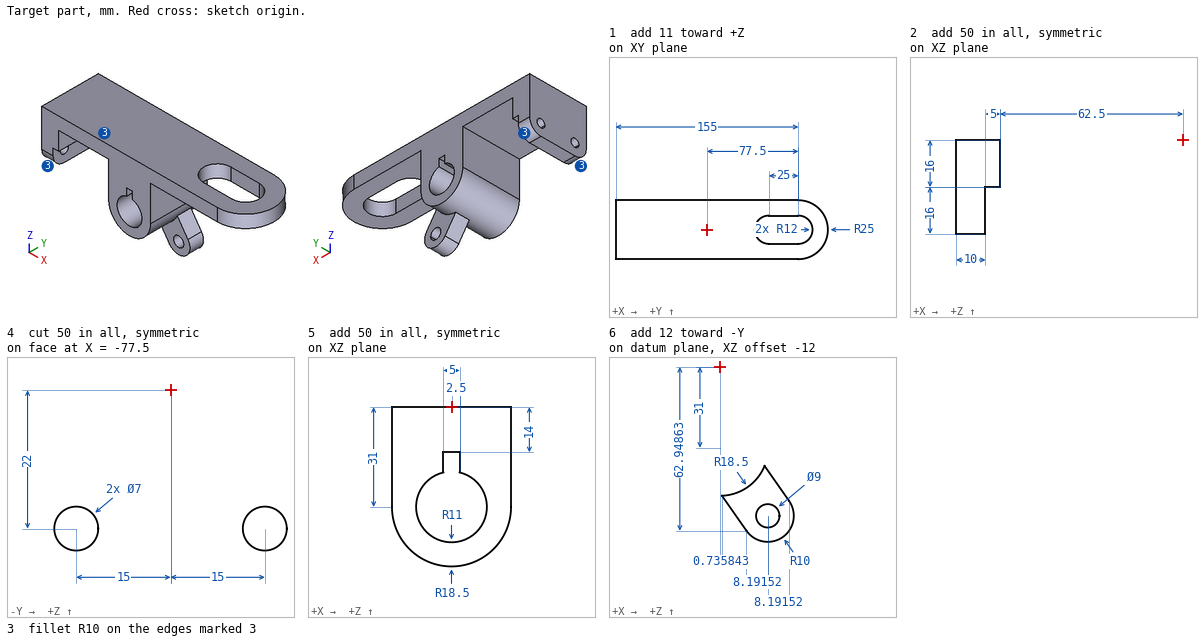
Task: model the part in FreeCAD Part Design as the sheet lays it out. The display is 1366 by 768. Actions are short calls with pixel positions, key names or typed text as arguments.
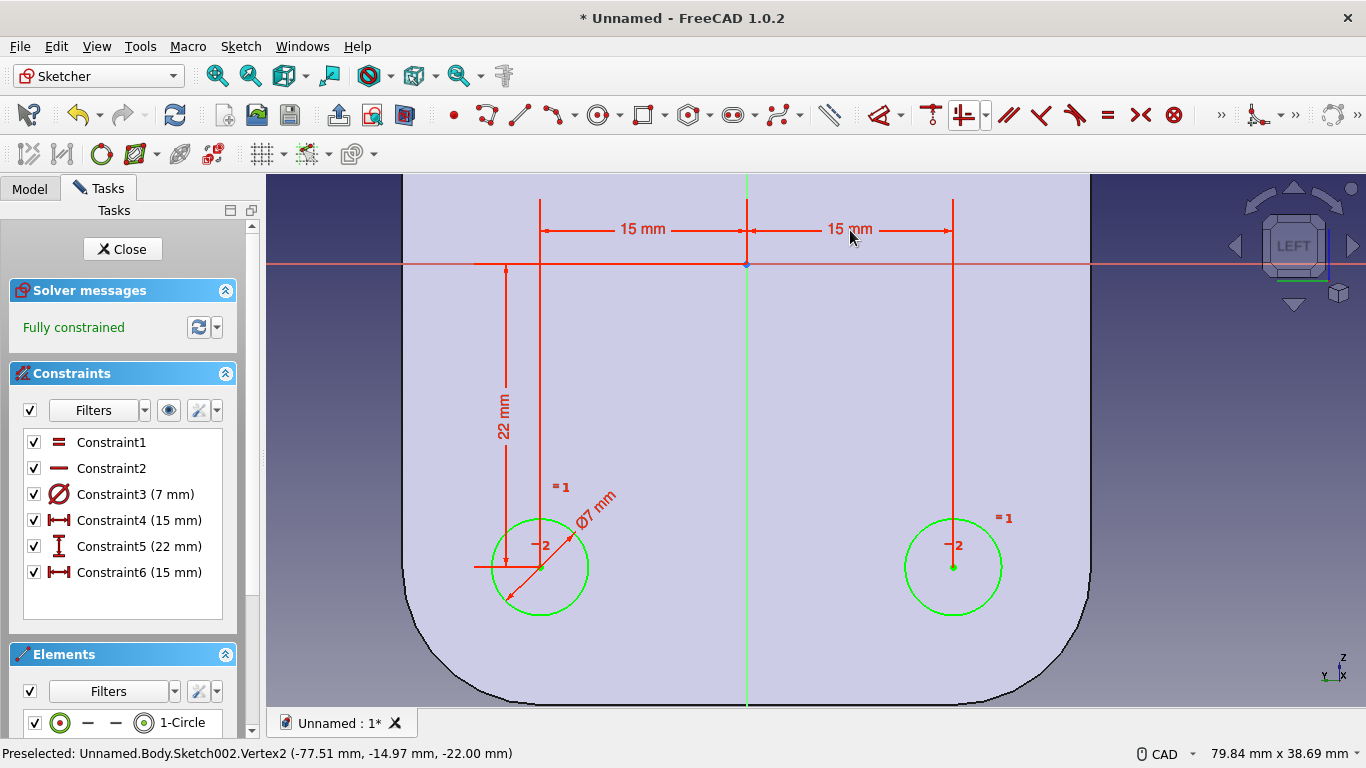
click(123, 249)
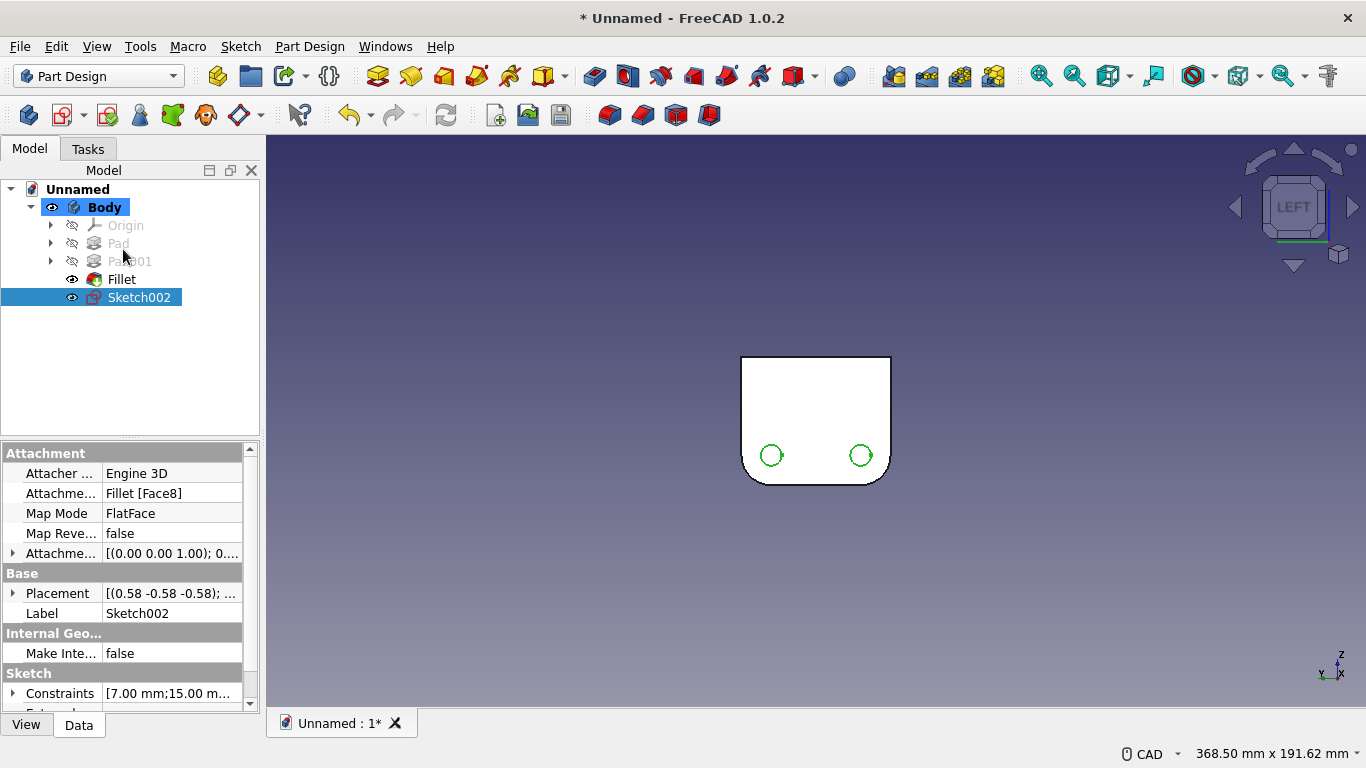
click(595, 76)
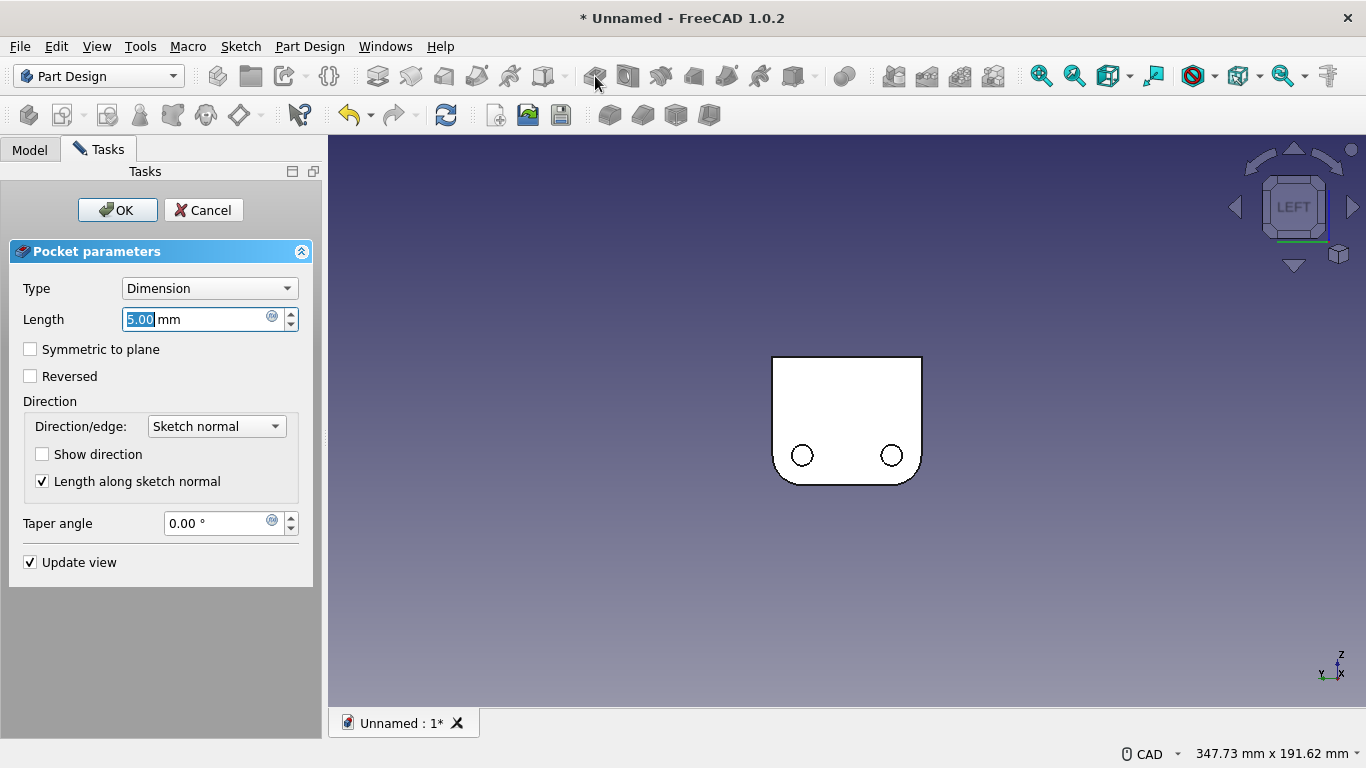
text(50)
key(Tab)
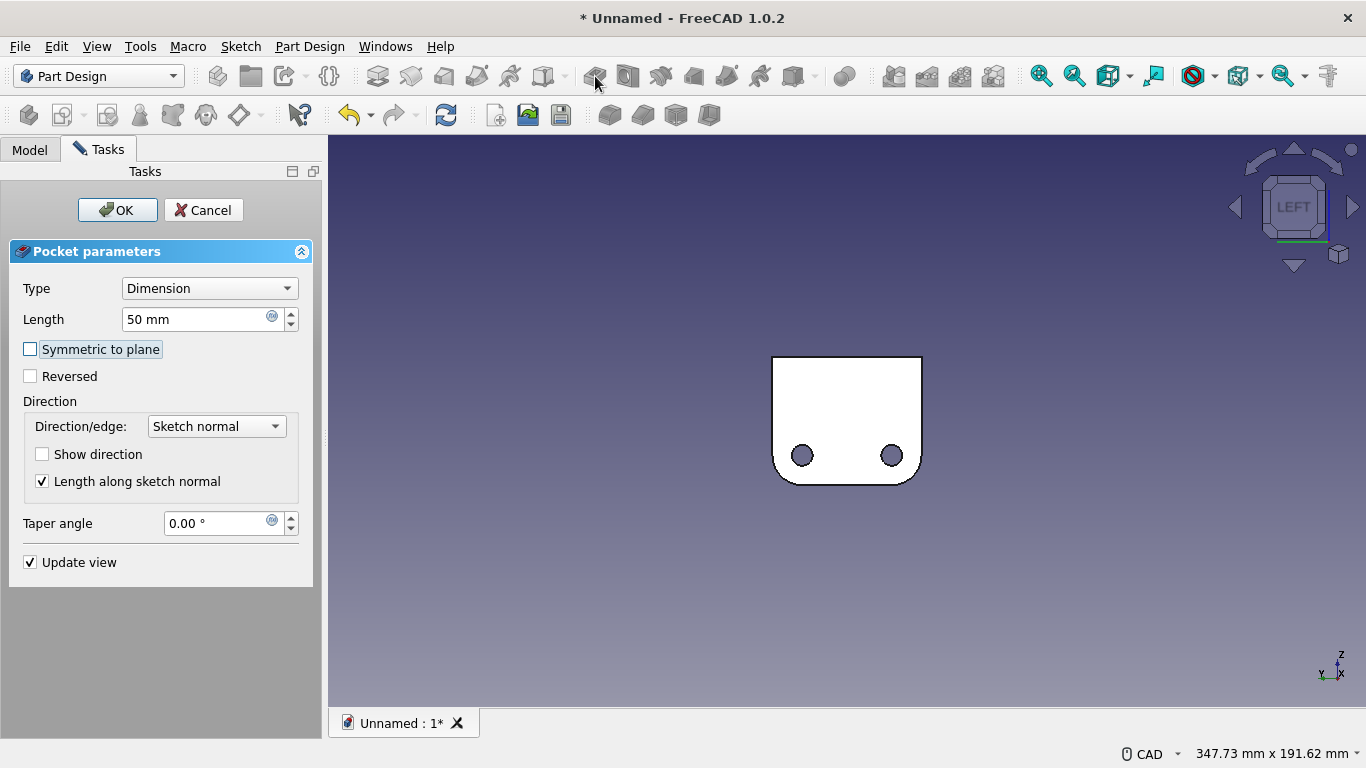
click(31, 349)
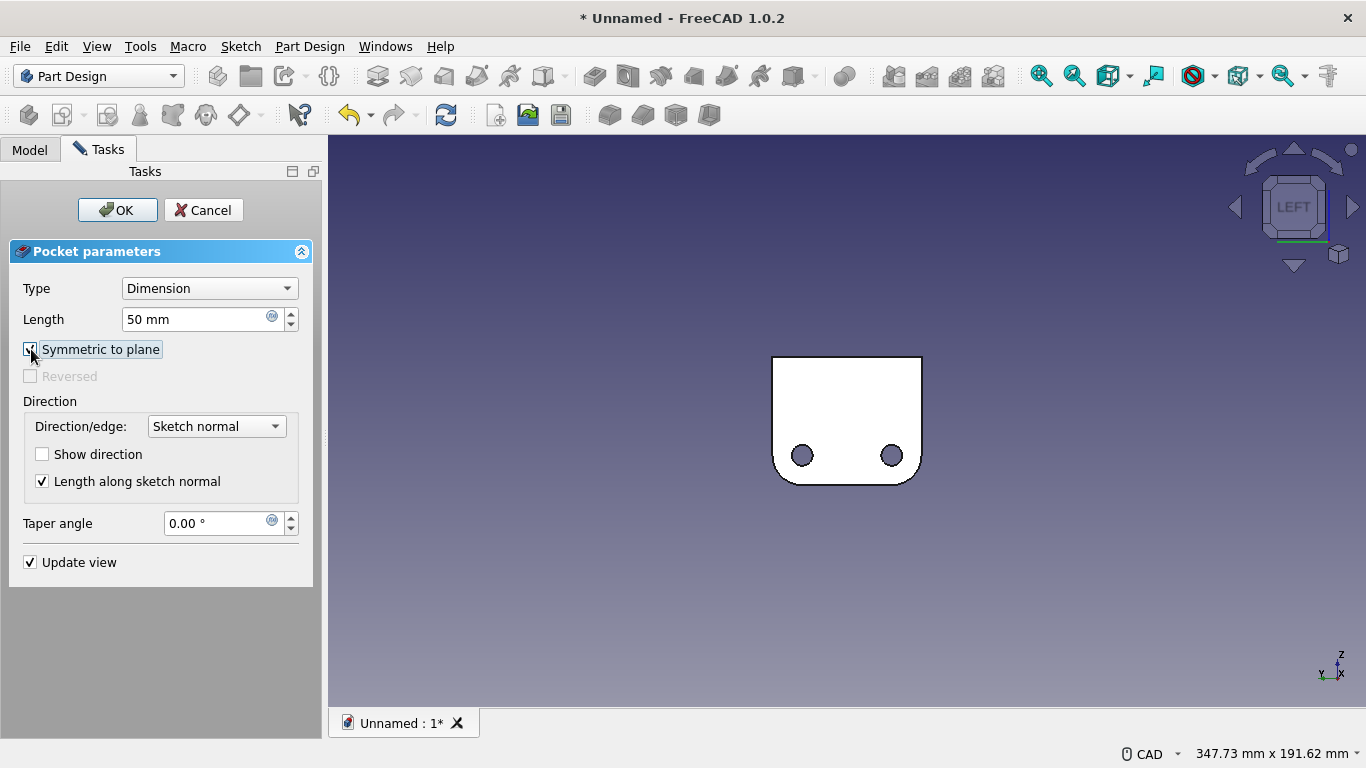
click(118, 210)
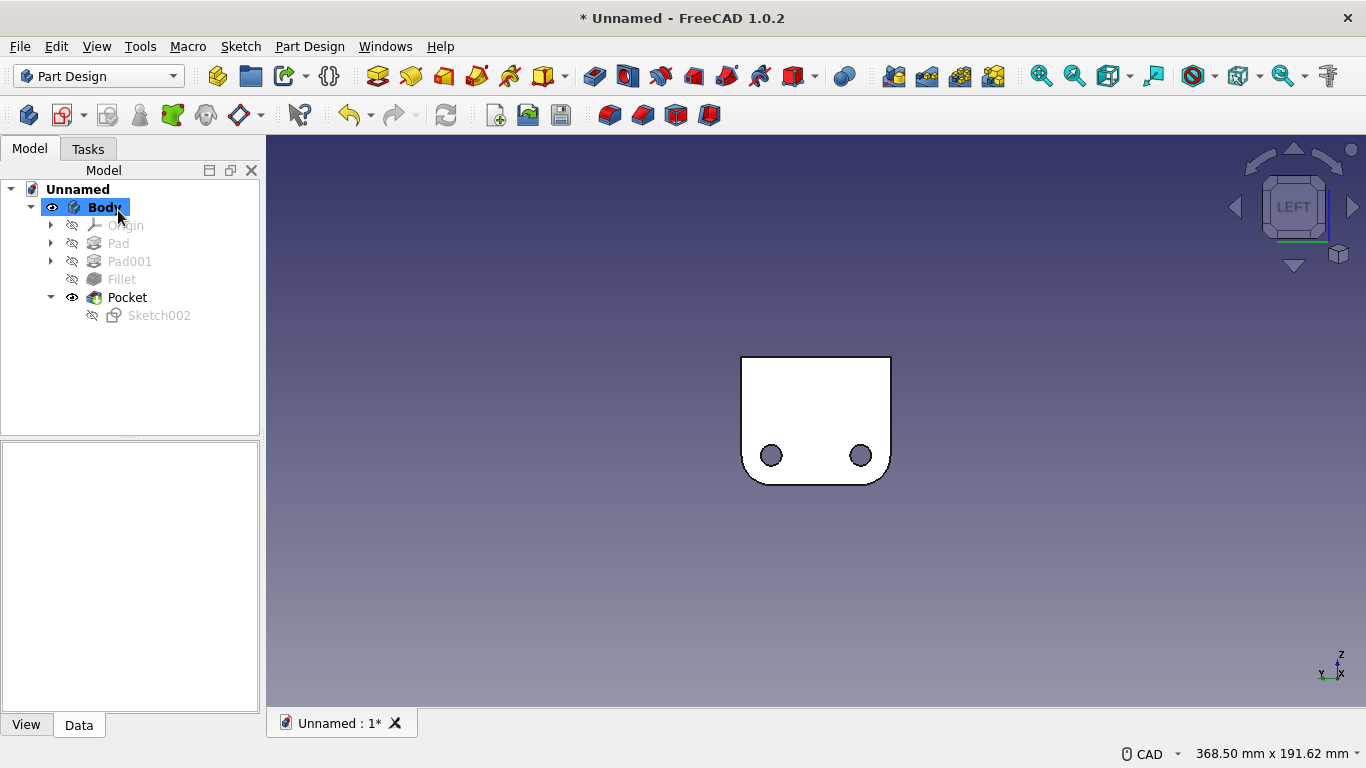
click(1042, 76)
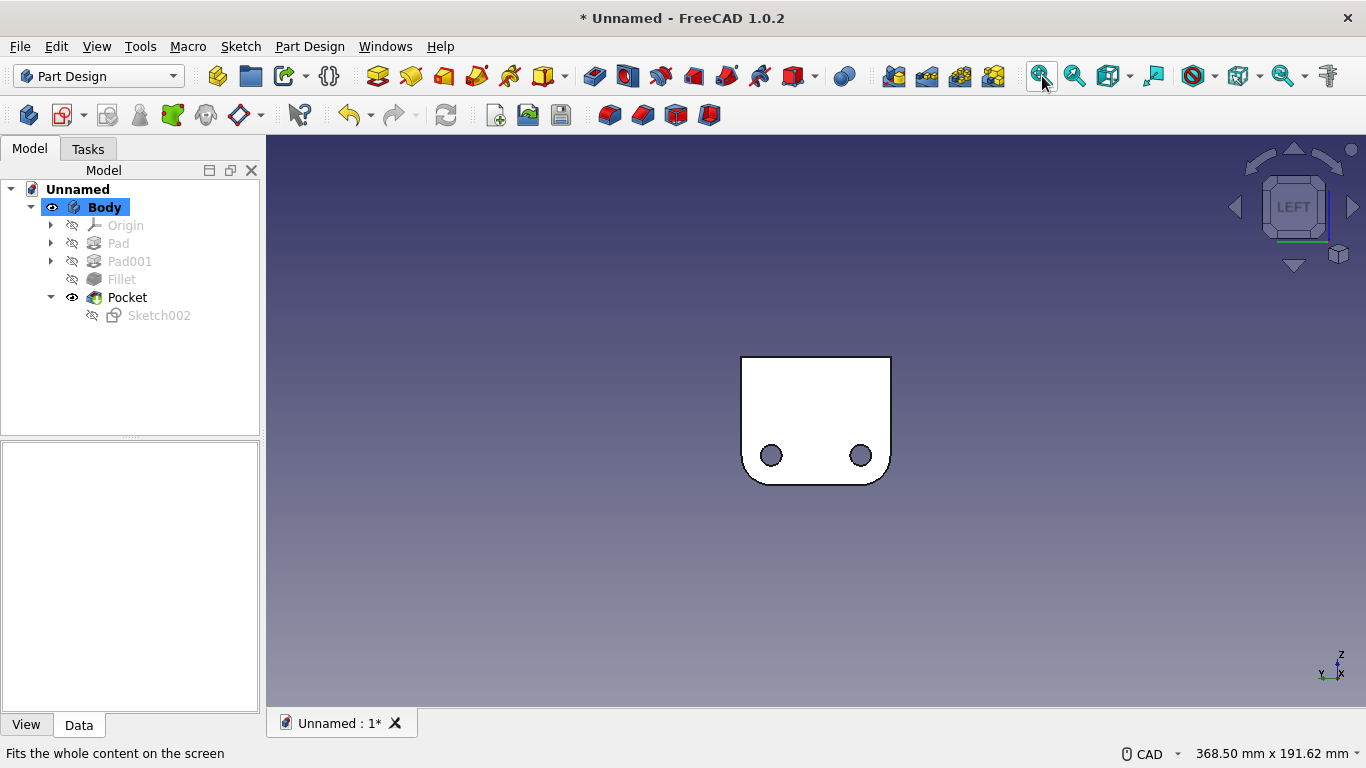
click(62, 116)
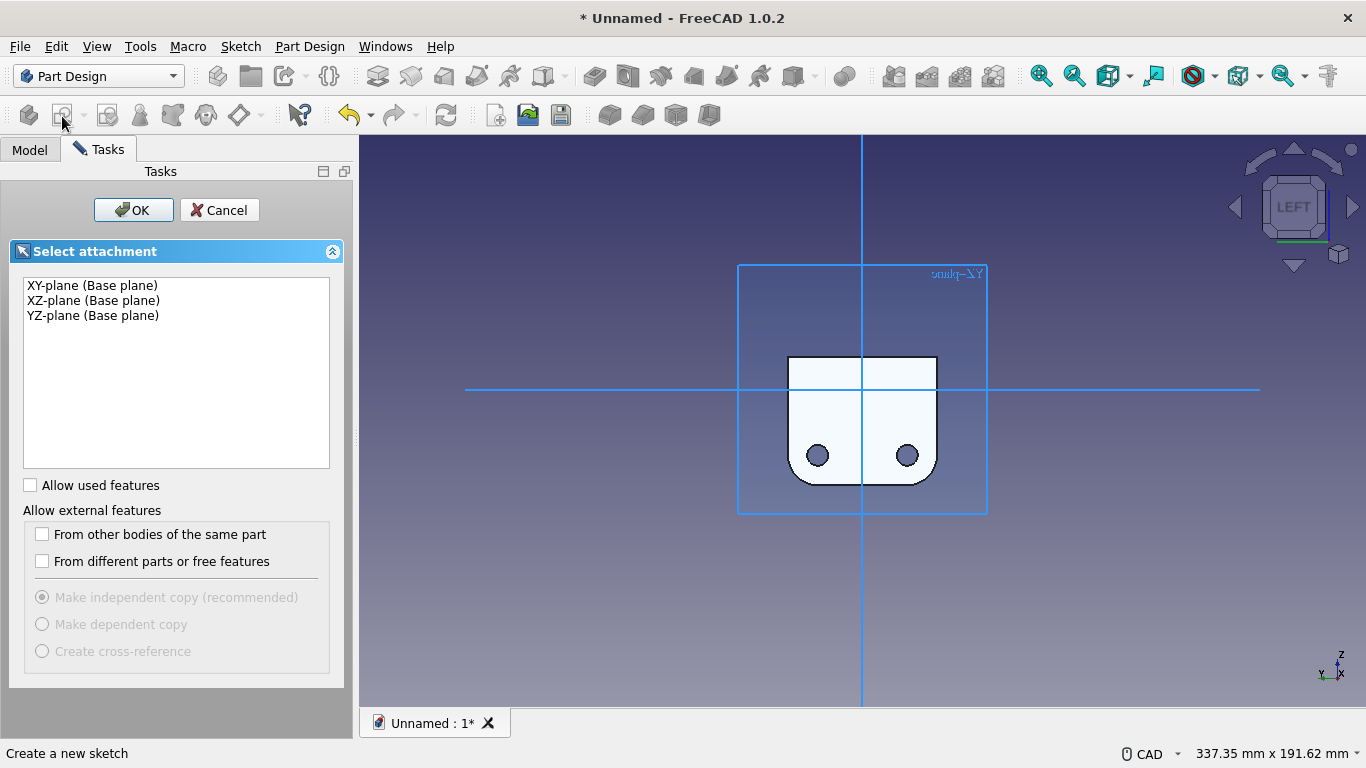
click(84, 300)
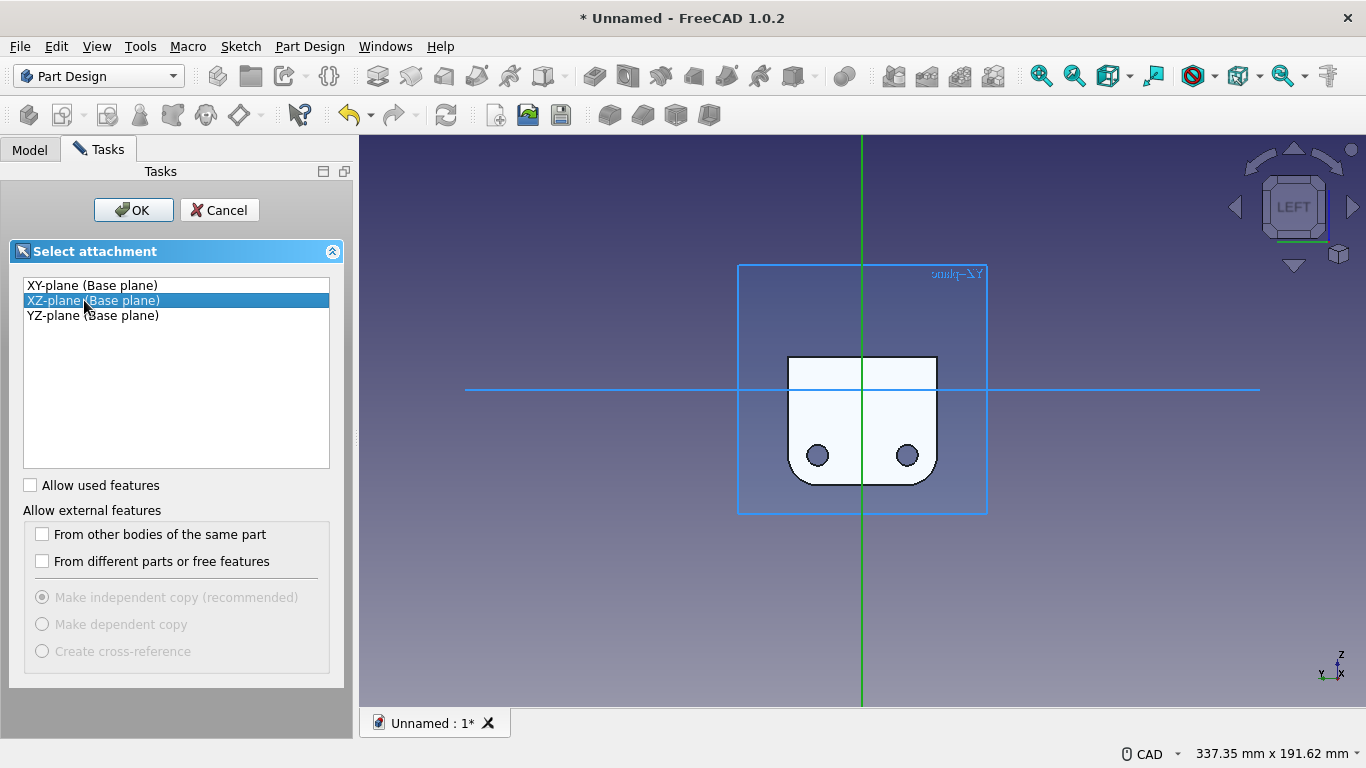
click(134, 210)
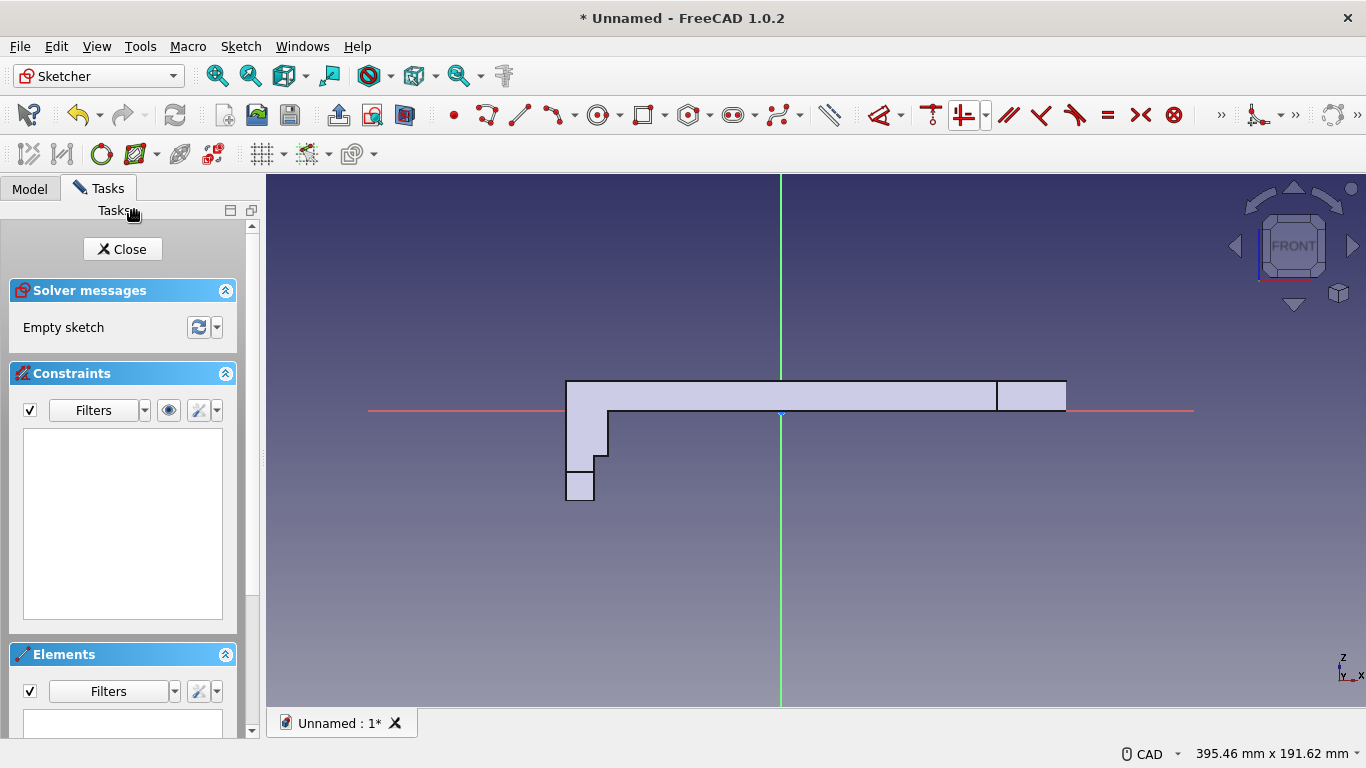
click(405, 116)